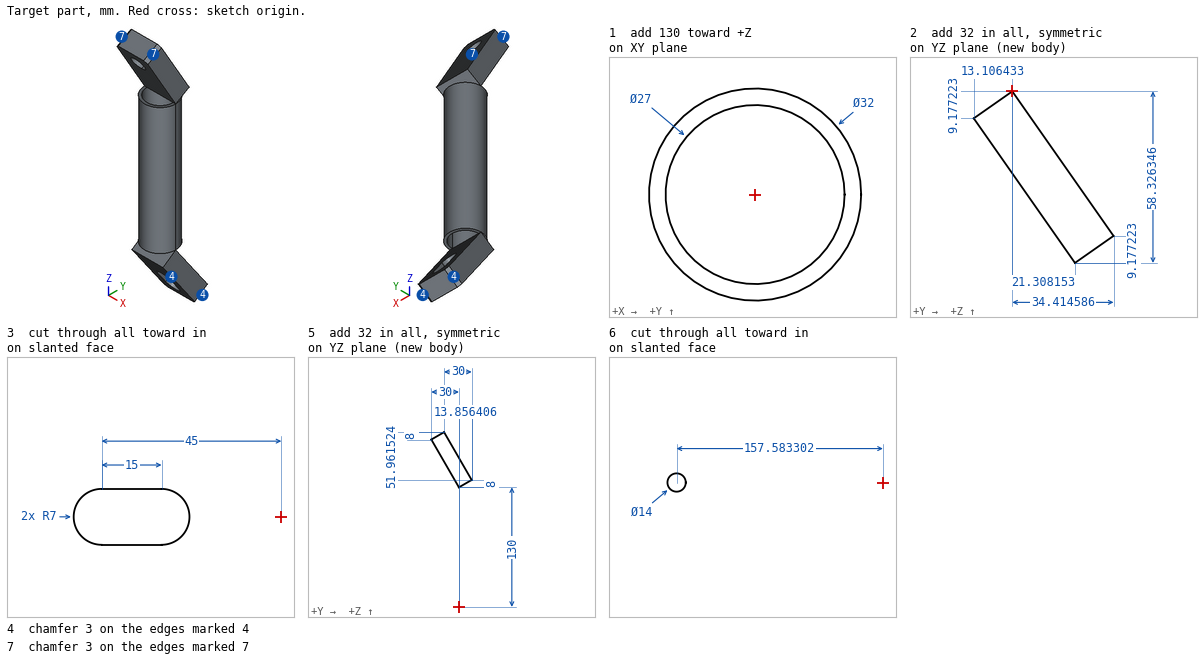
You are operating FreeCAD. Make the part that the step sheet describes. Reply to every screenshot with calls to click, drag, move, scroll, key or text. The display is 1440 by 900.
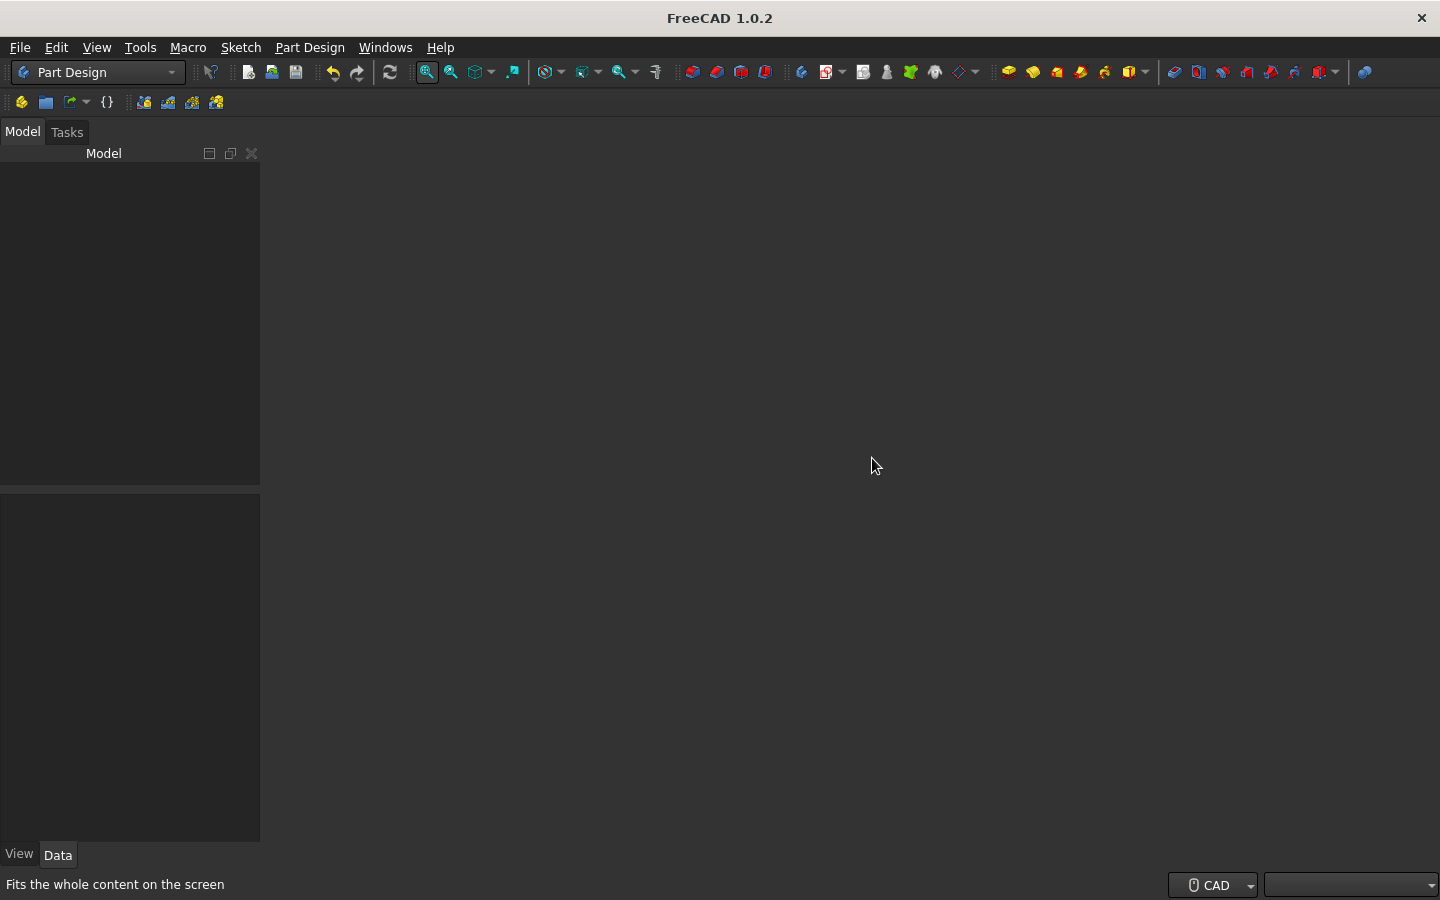
key(ctrl+n)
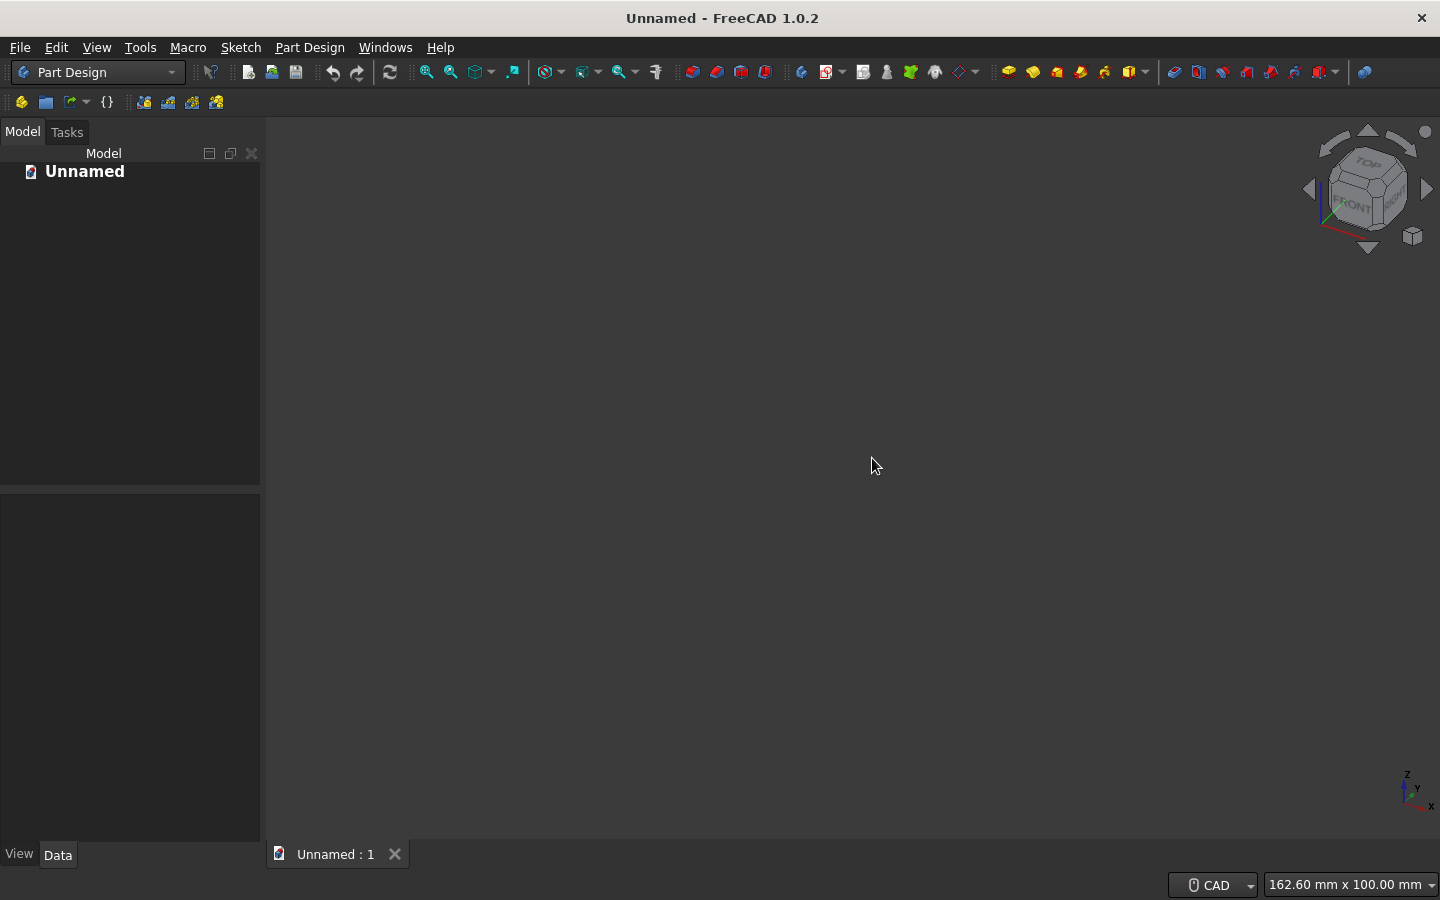
click(826, 72)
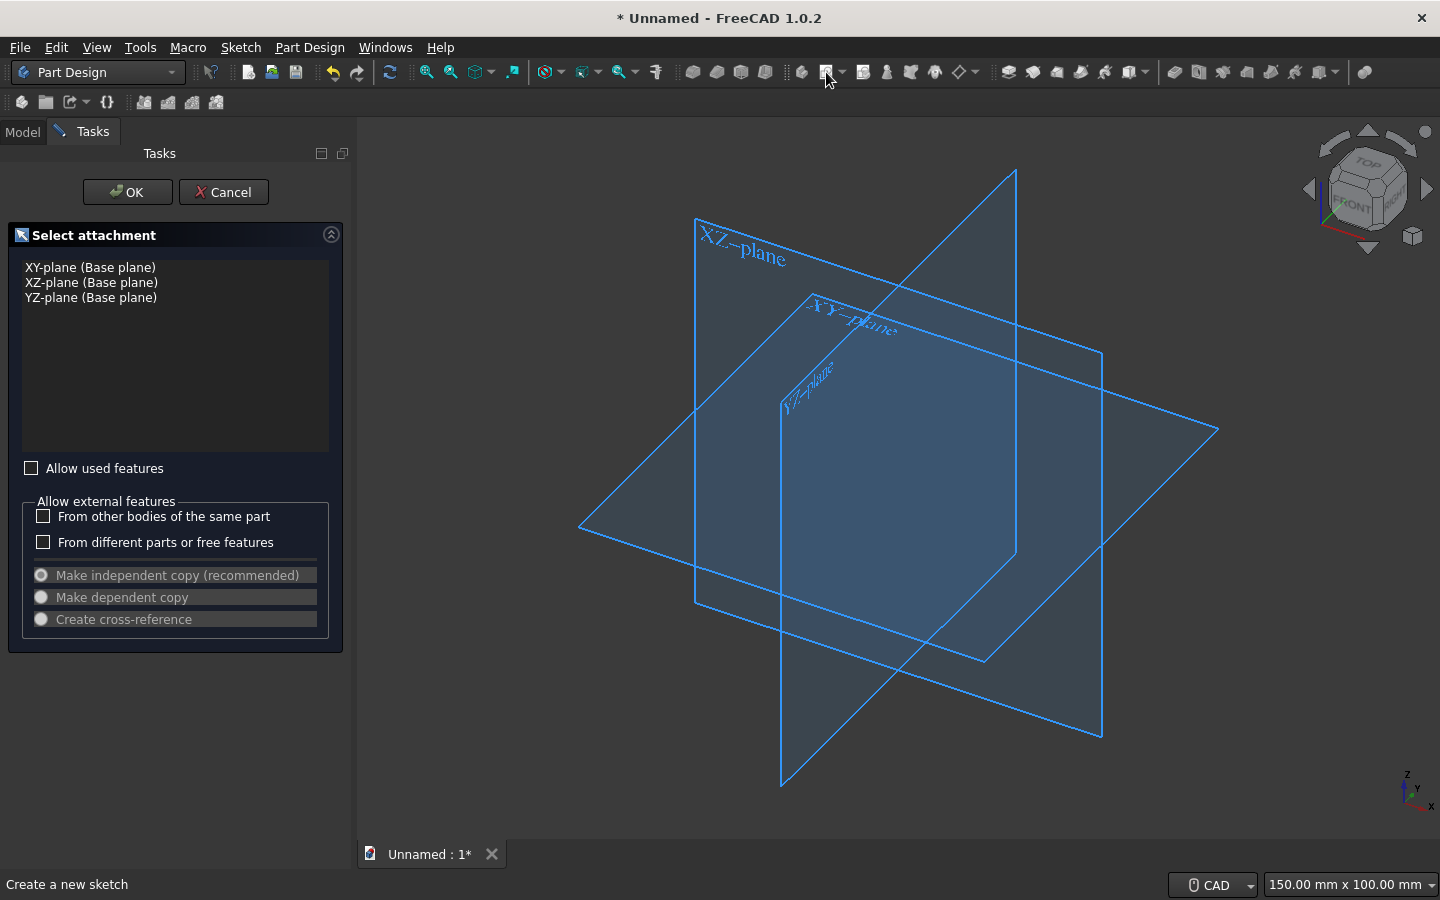
click(82, 268)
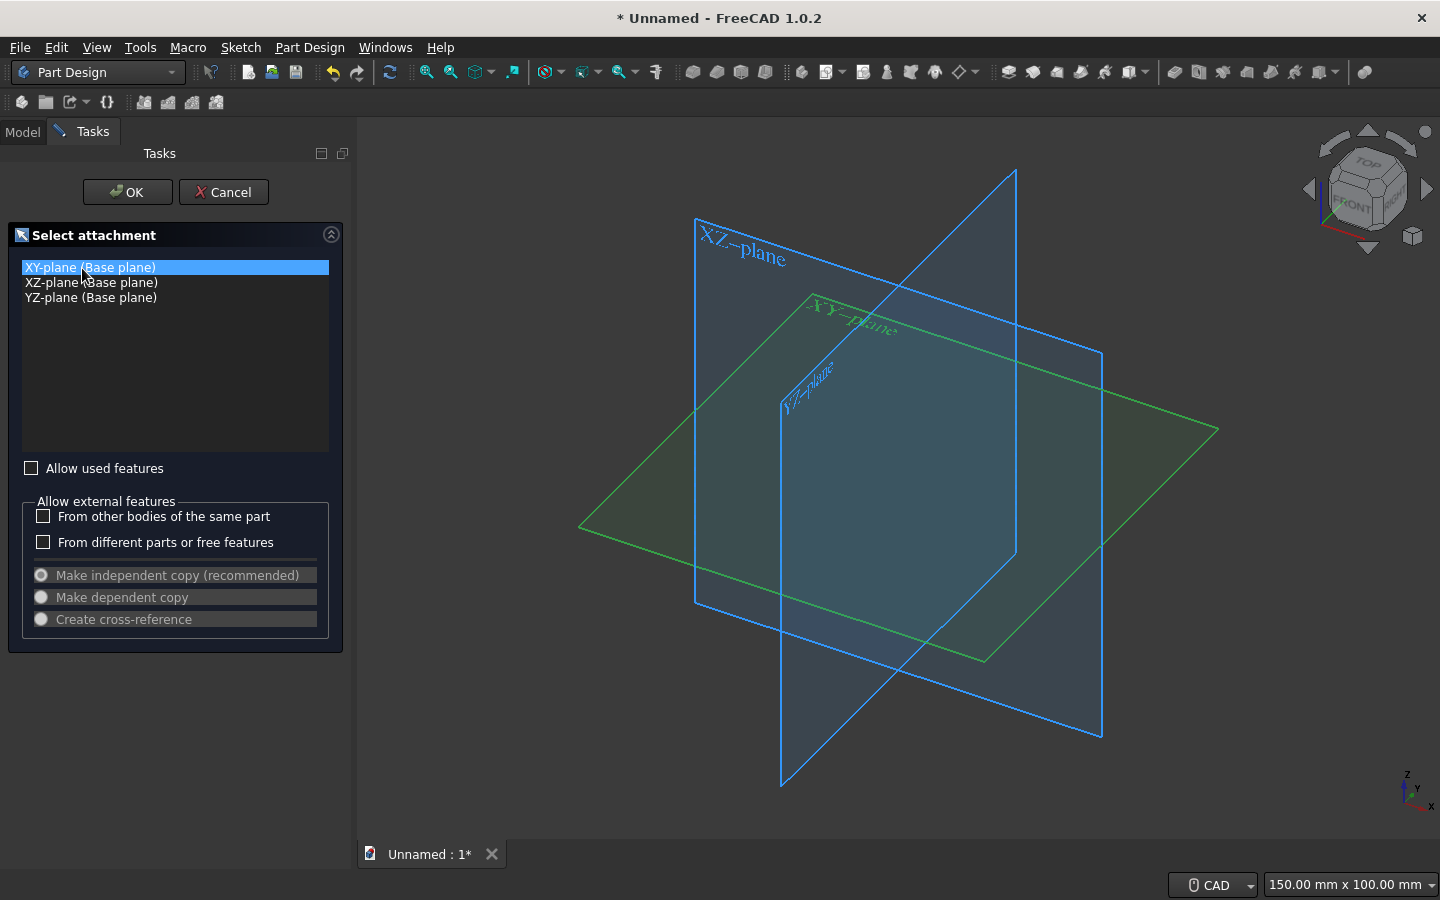
click(128, 192)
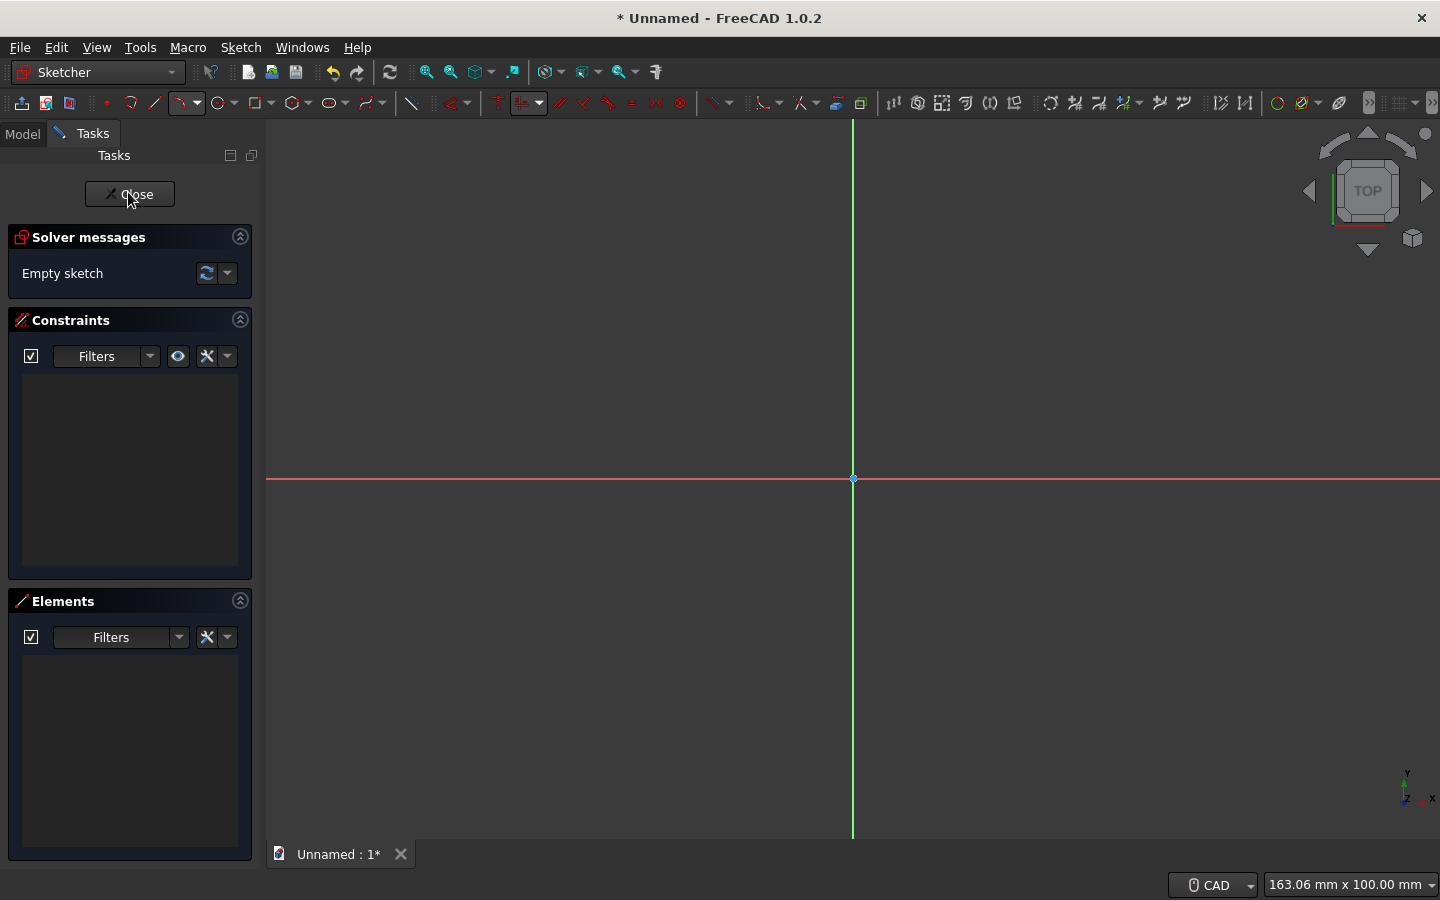
scroll(909, 479, up, 4)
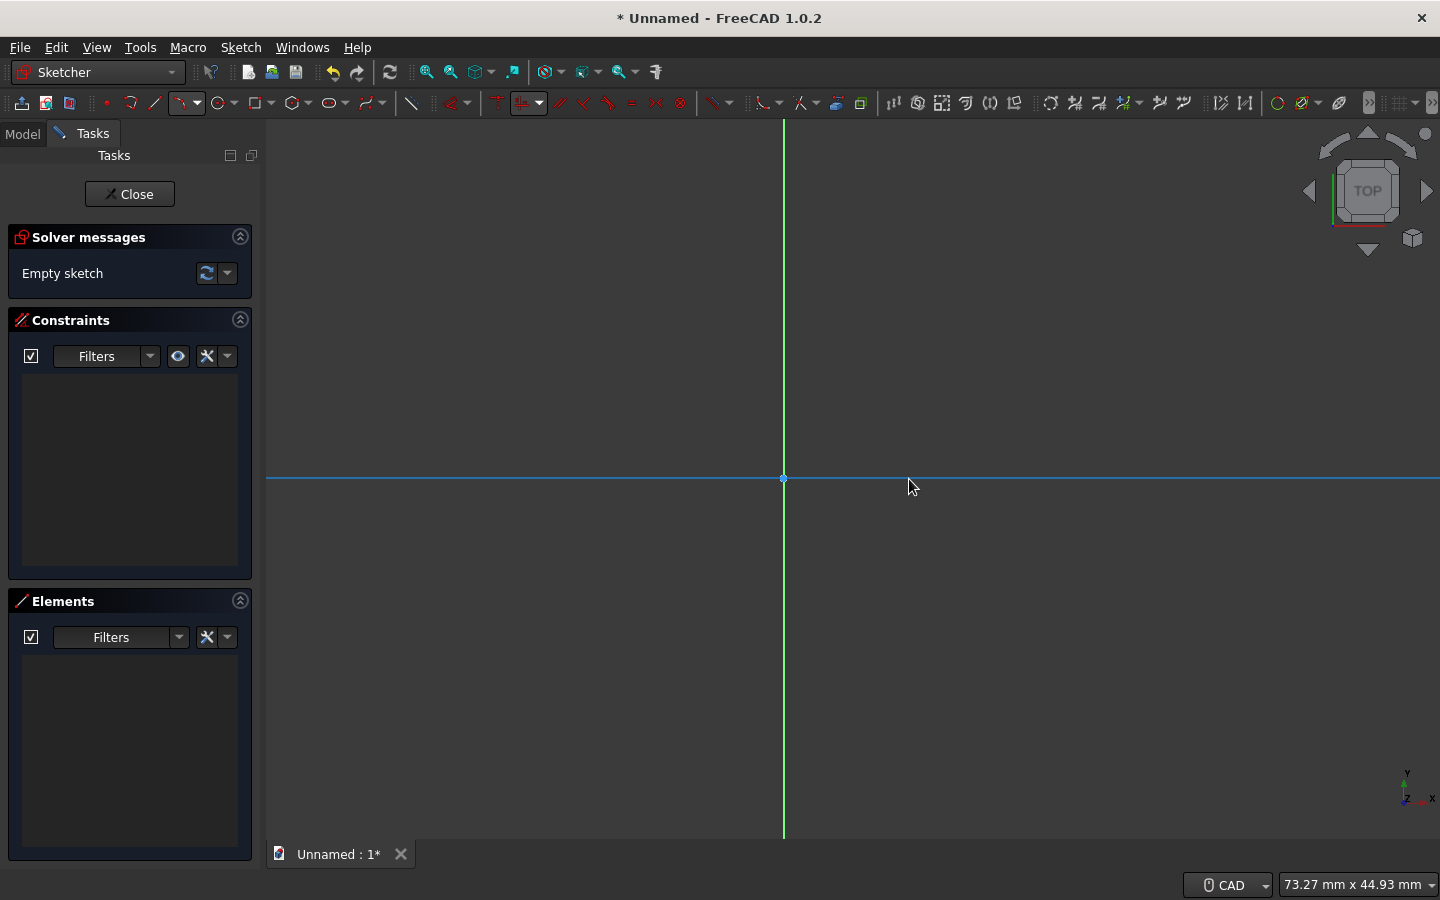
key(g)
key(c)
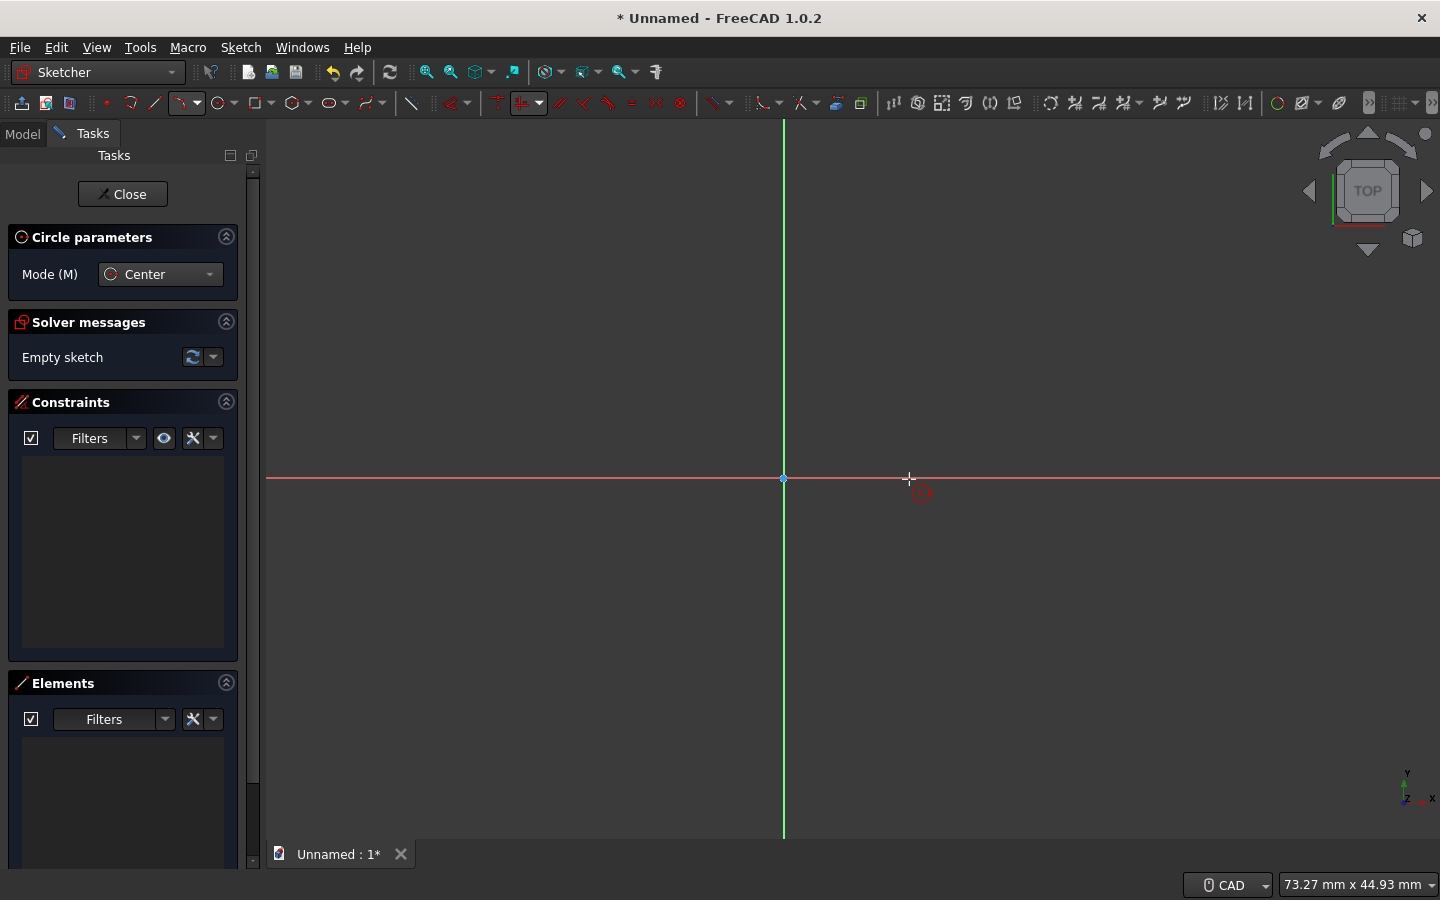
click(784, 478)
click(965, 297)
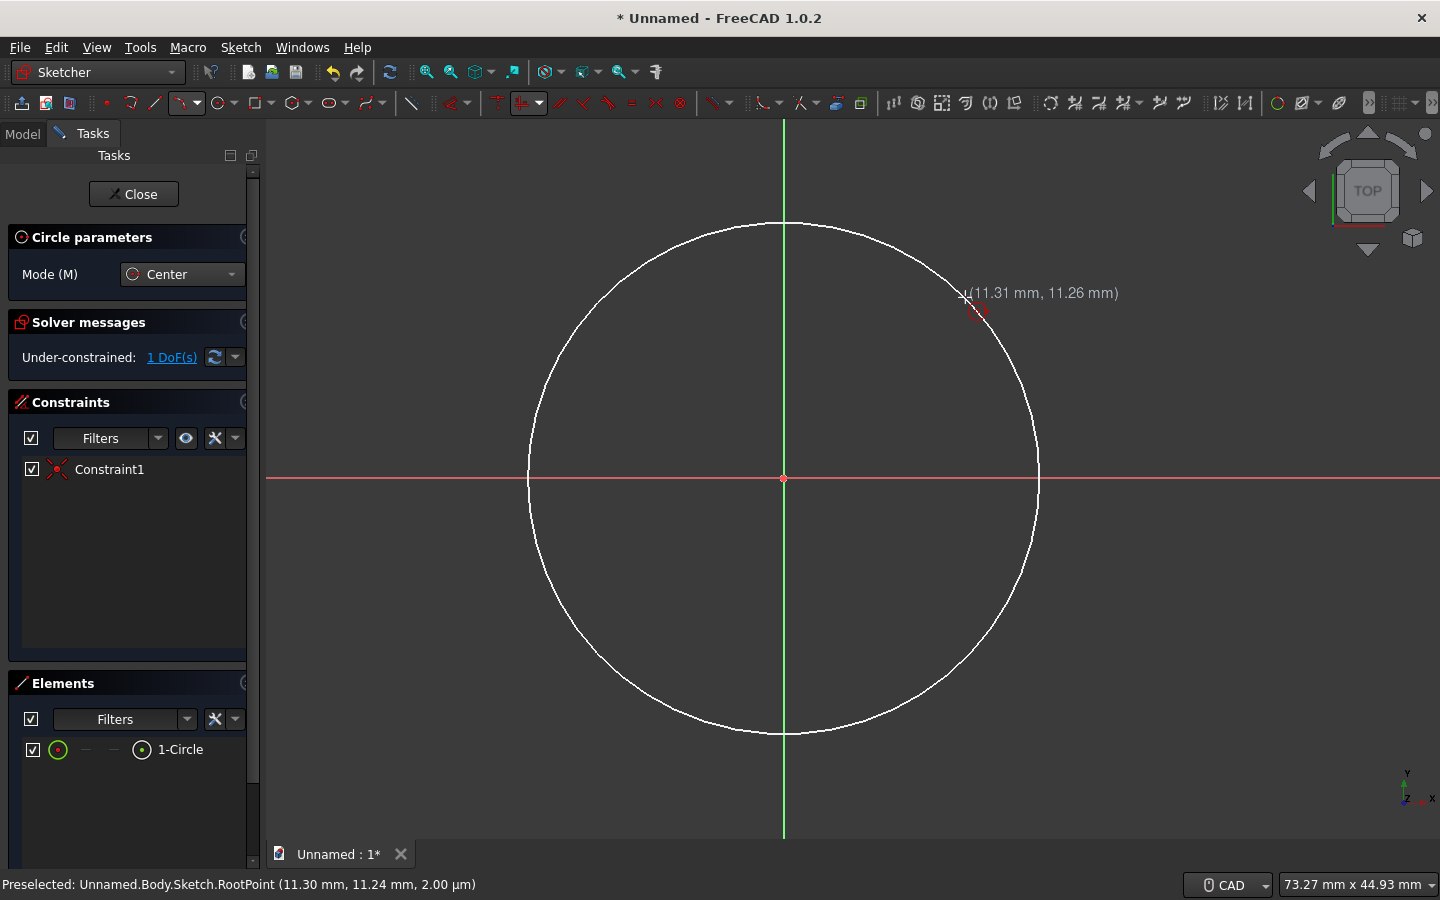
click(784, 478)
click(937, 325)
key(Escape)